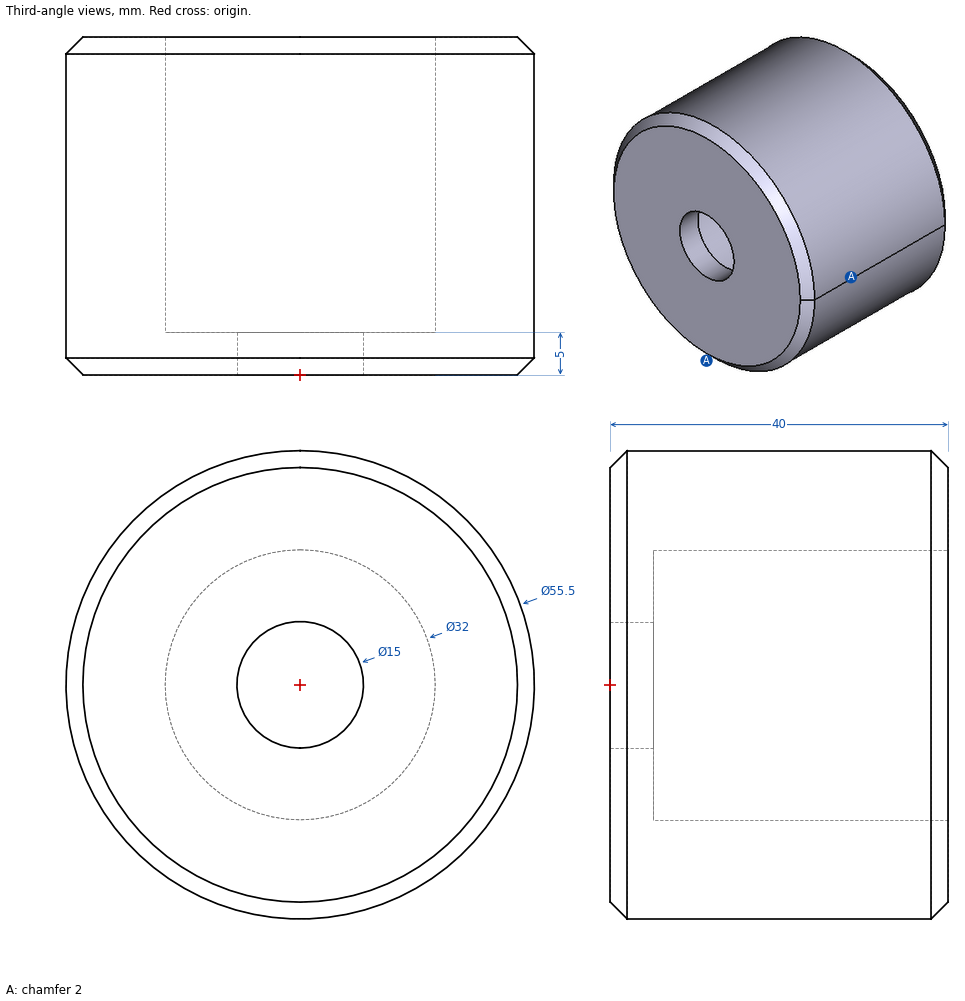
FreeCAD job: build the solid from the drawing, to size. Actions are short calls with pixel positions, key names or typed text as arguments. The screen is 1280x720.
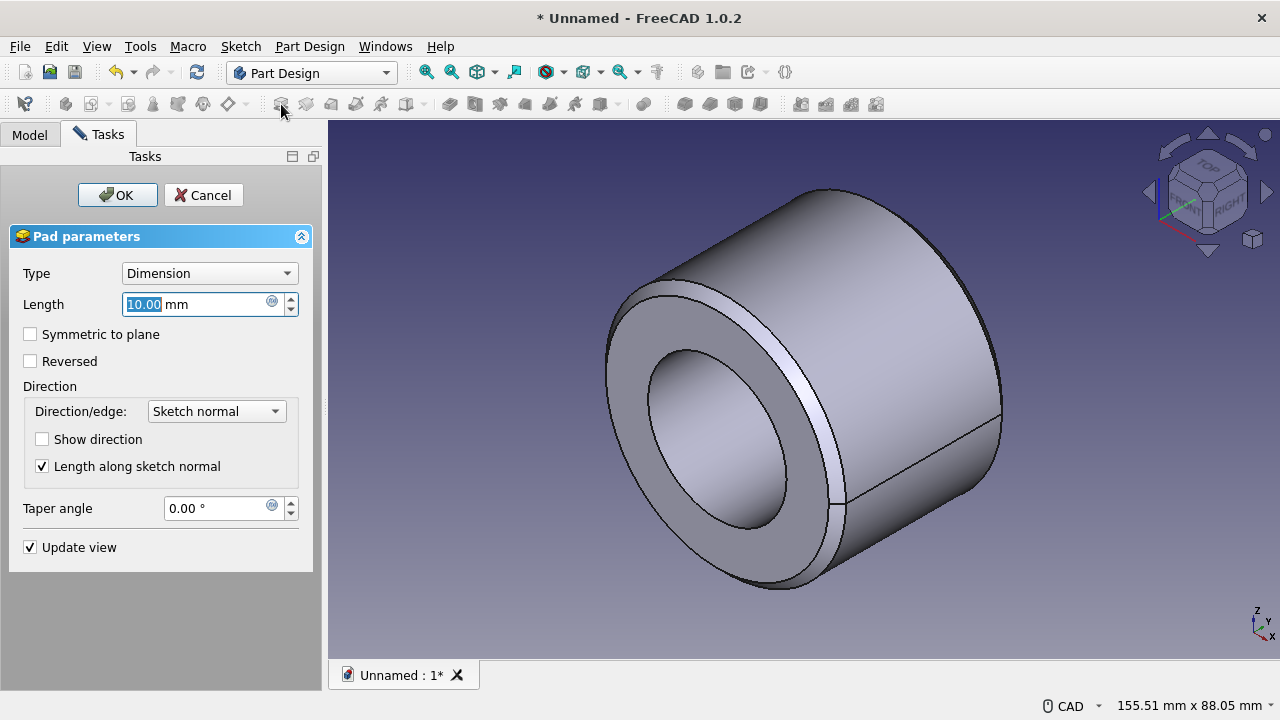
text(5)
key(Tab)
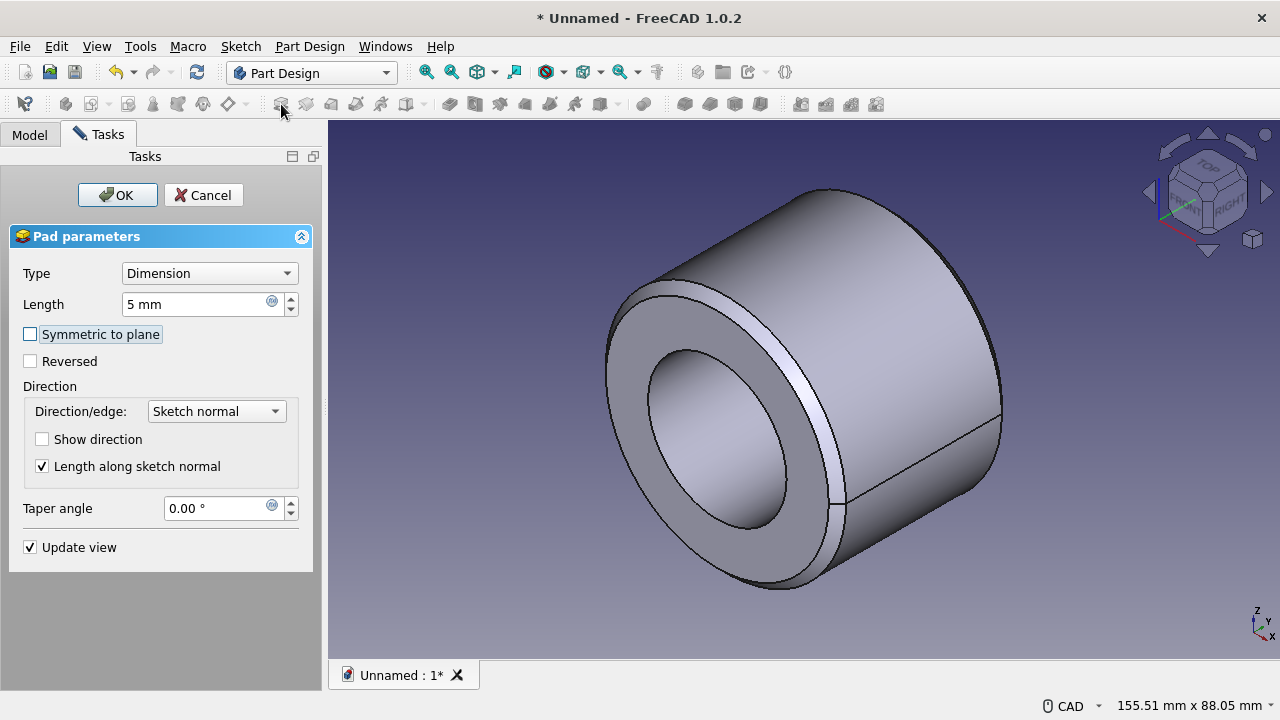
click(31, 361)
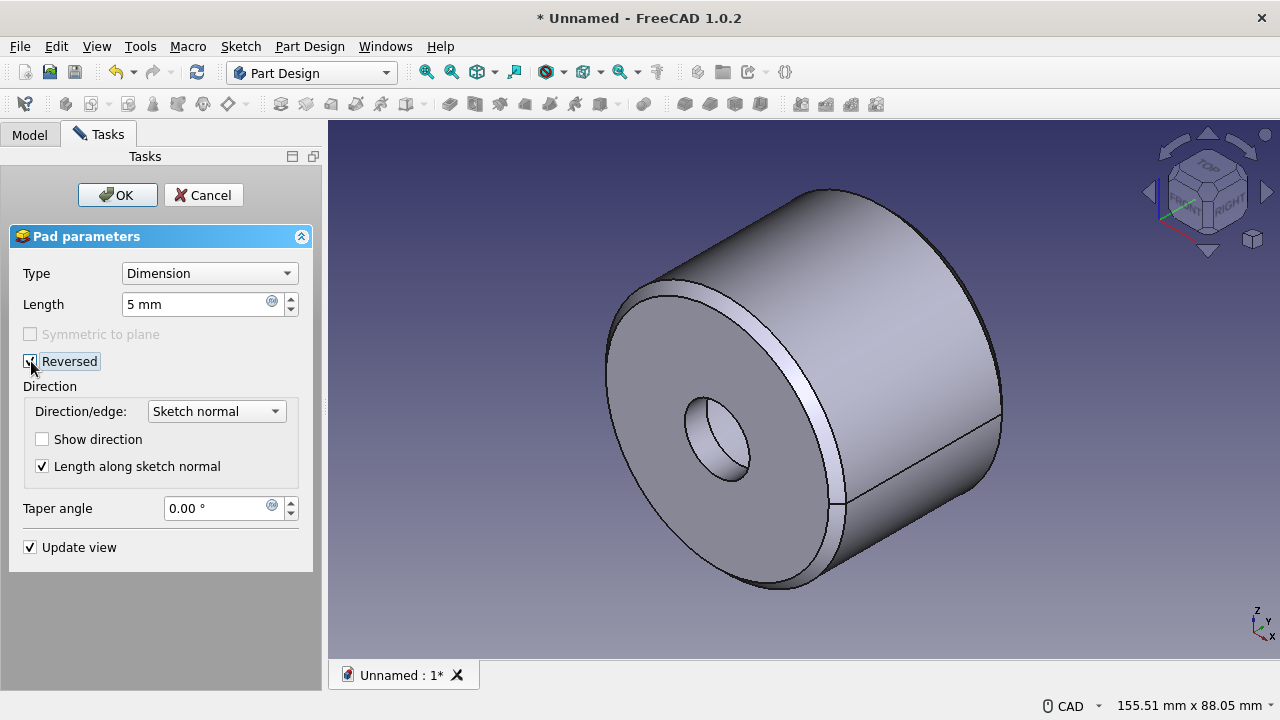
click(118, 195)